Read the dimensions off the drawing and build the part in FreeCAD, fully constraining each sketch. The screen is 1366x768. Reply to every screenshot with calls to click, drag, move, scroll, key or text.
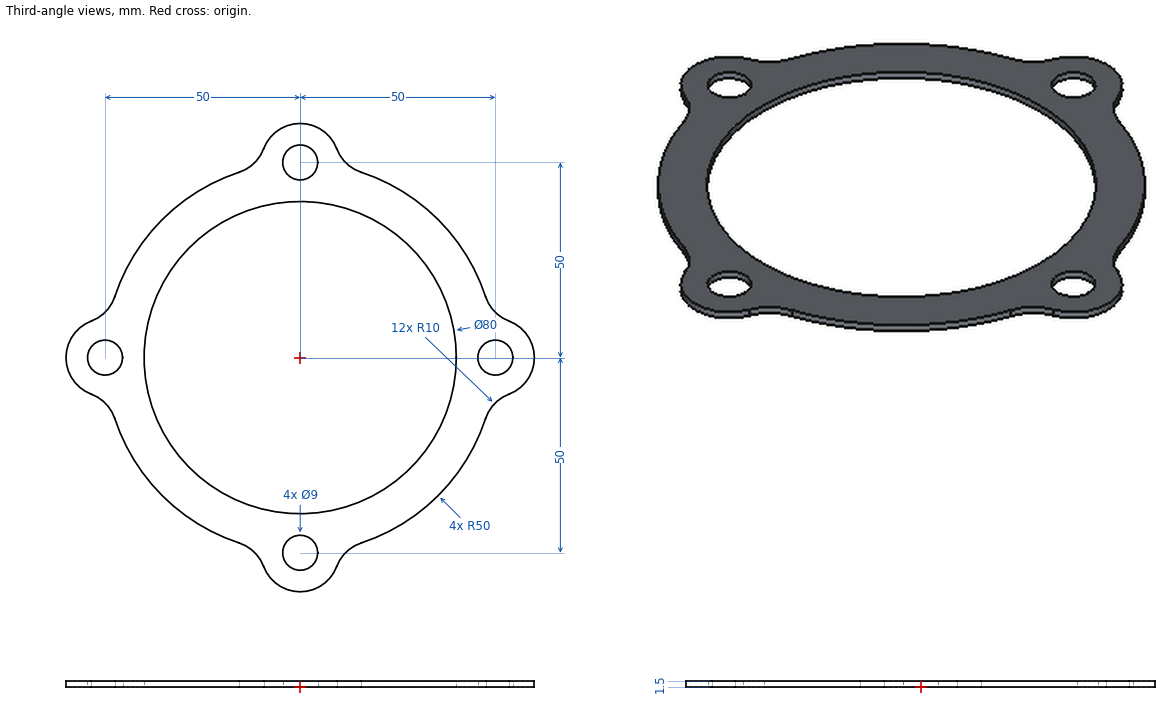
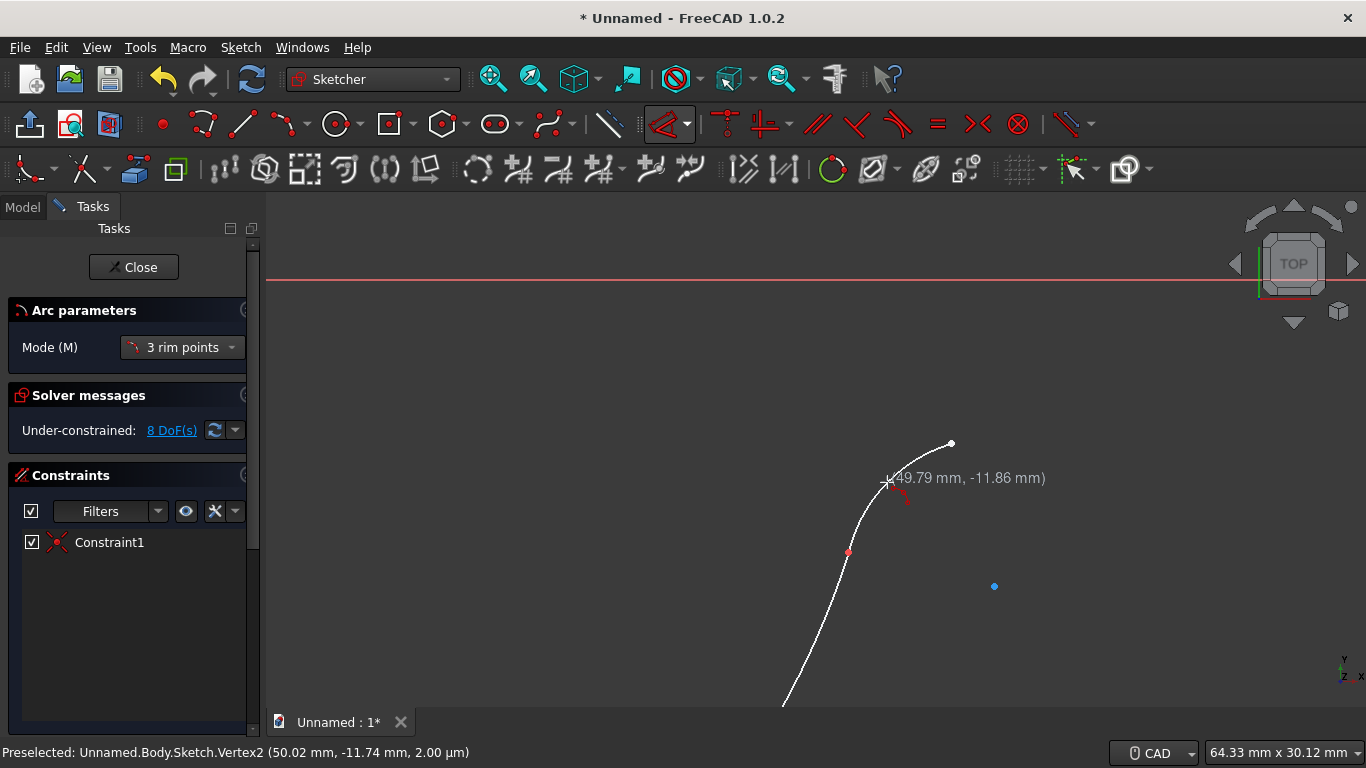
scroll(888, 483, down, 9)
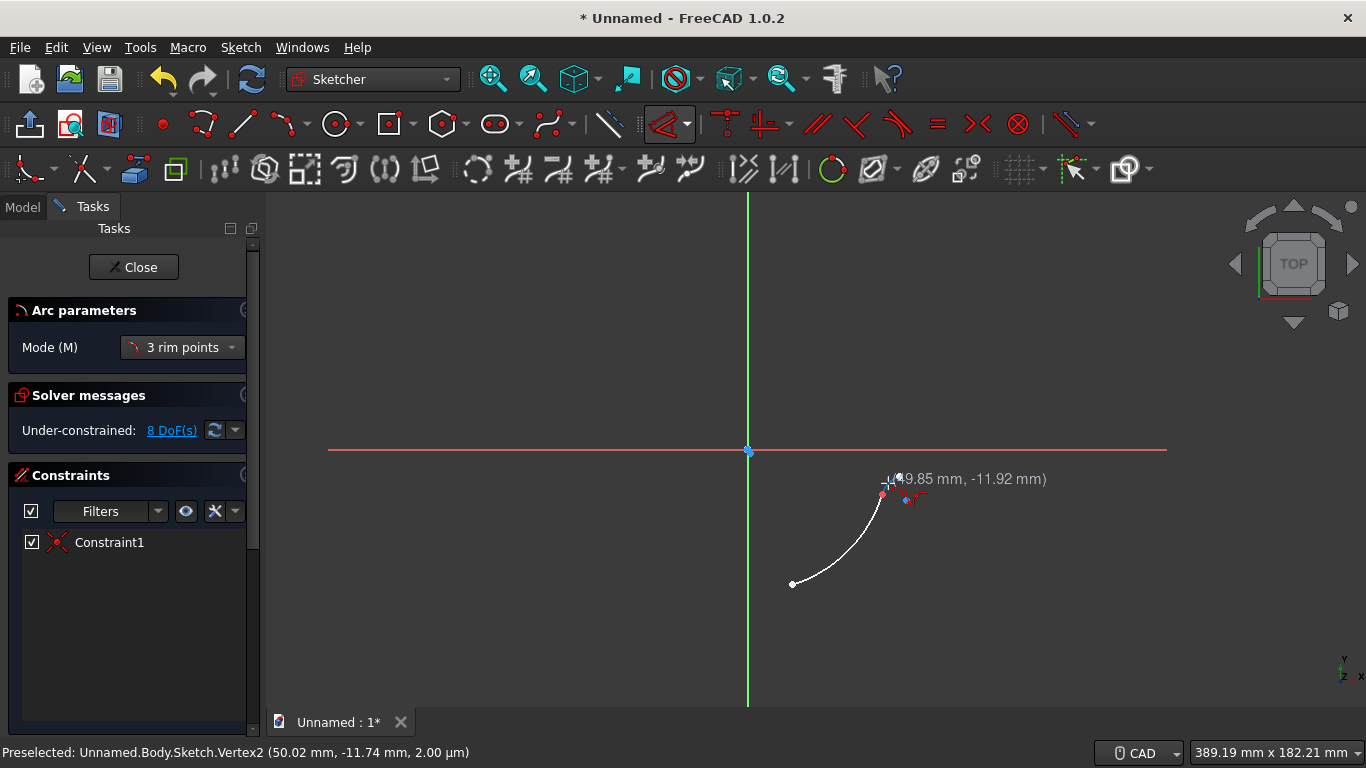
click(899, 477)
click(899, 423)
click(914, 463)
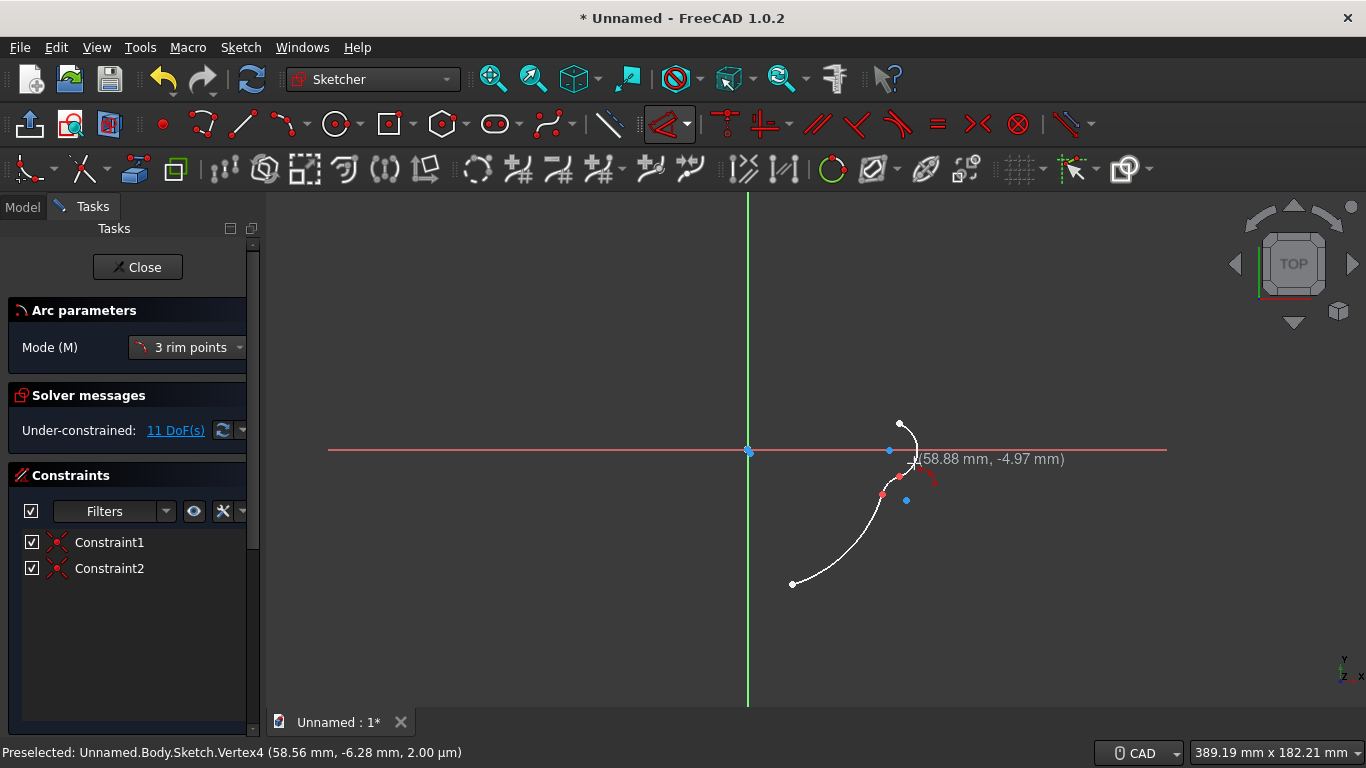
click(899, 424)
click(882, 406)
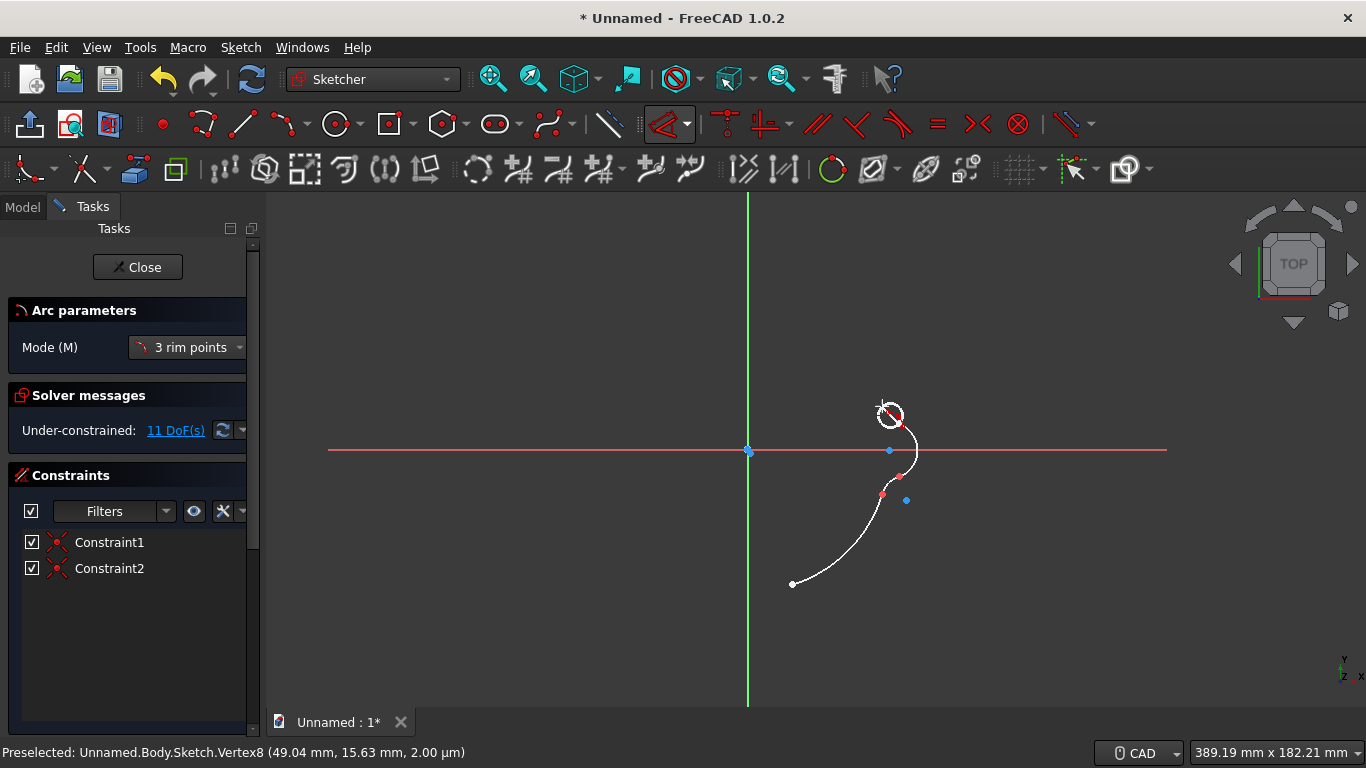
scroll(888, 417, up, 9)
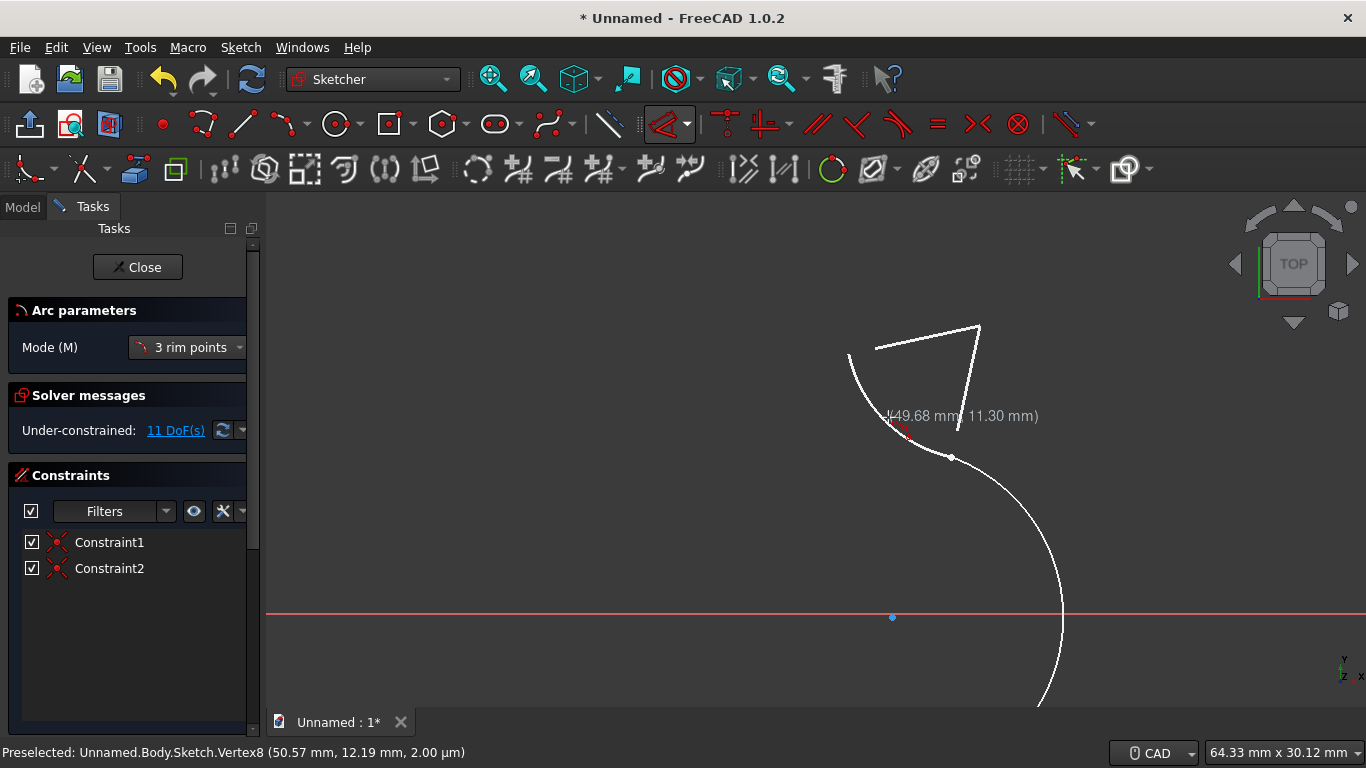
click(887, 412)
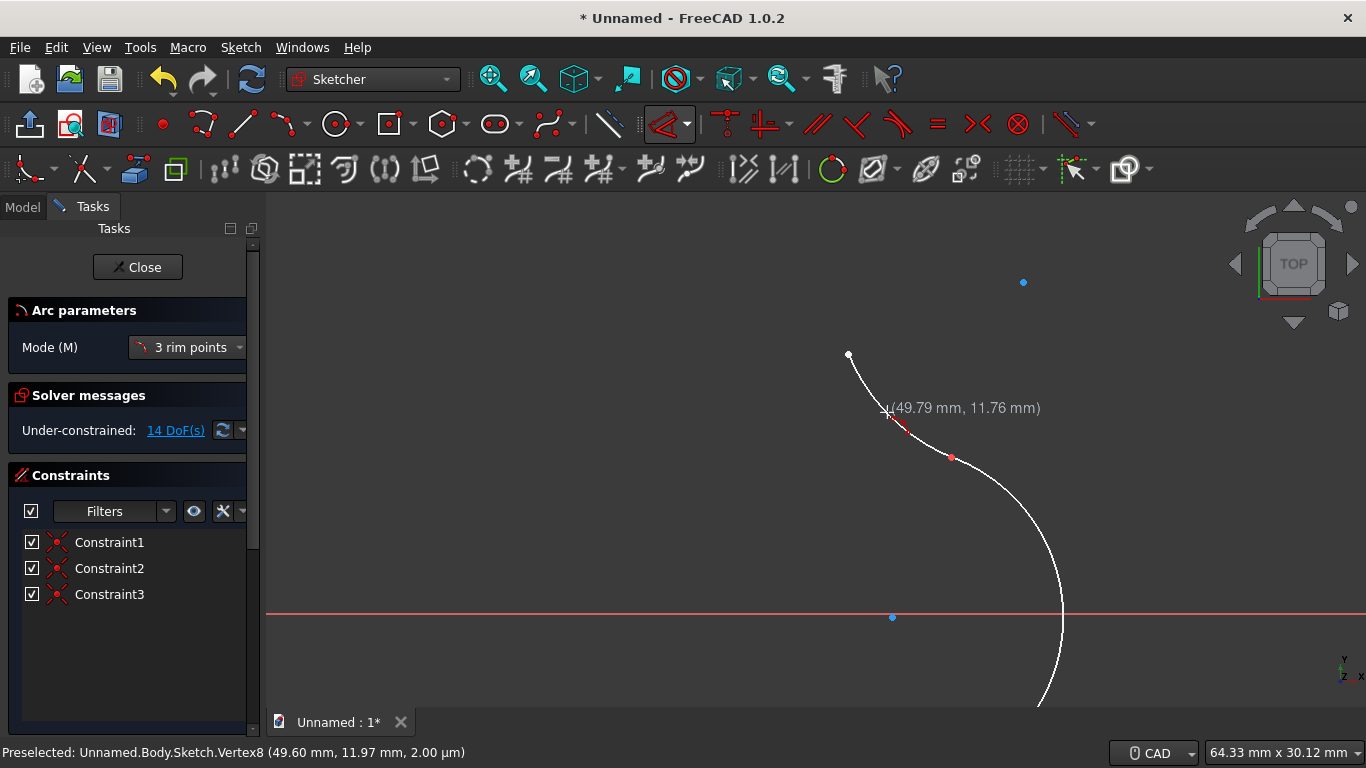
scroll(888, 417, down, 9)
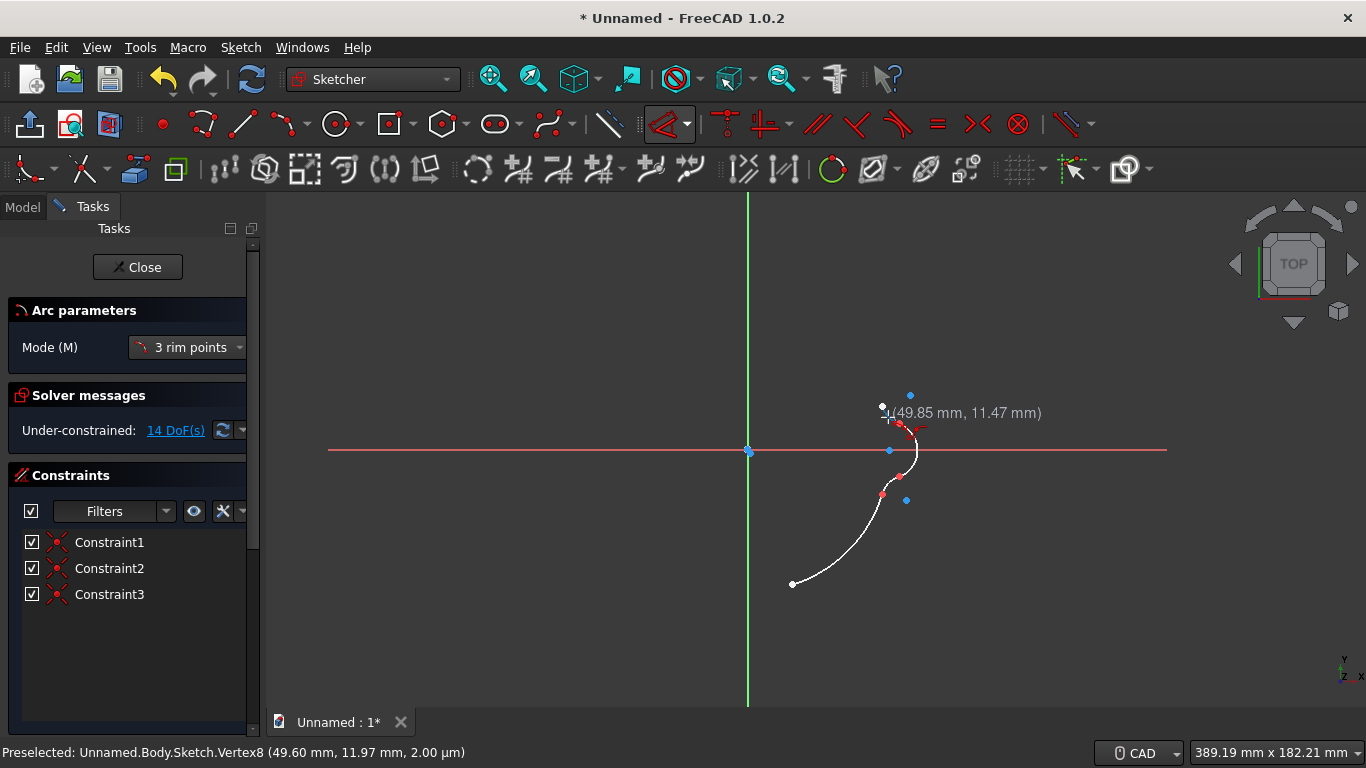
click(882, 407)
click(792, 316)
click(848, 350)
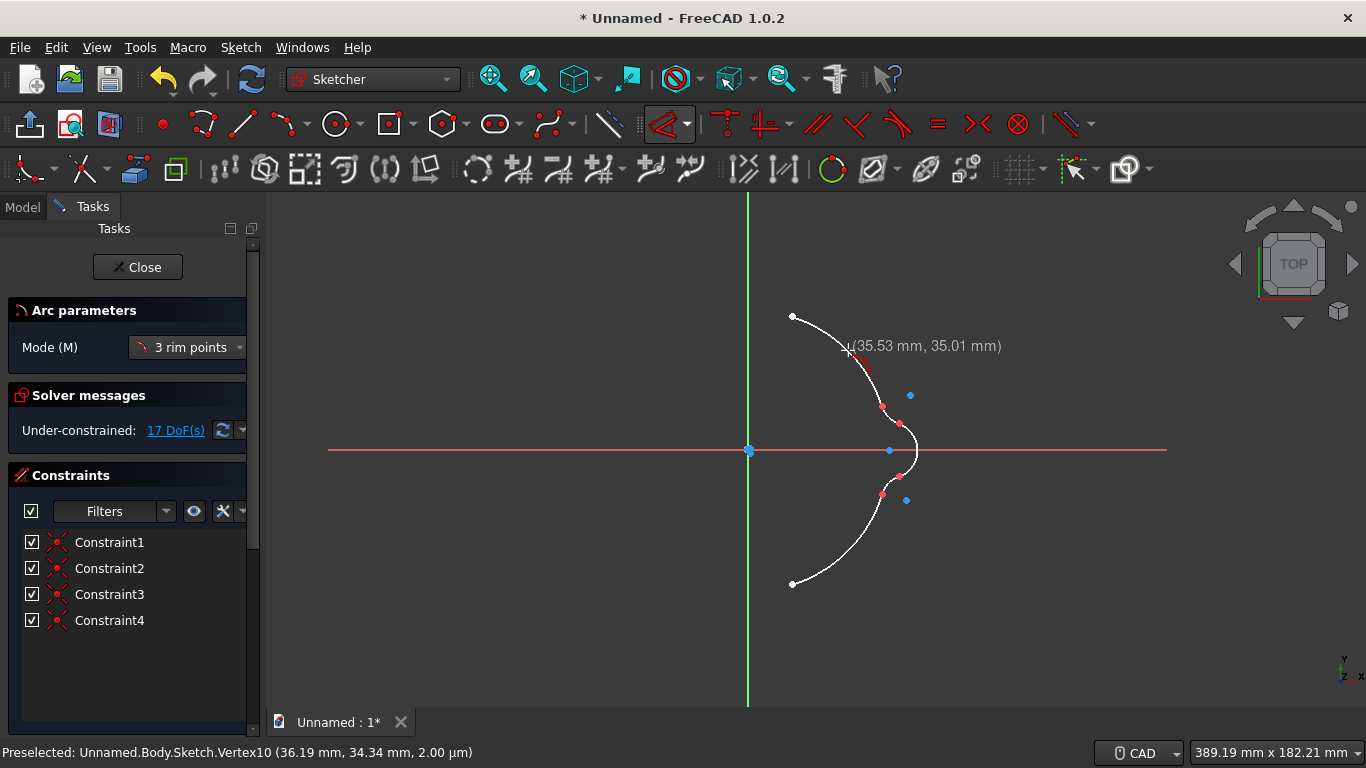
click(792, 317)
click(774, 299)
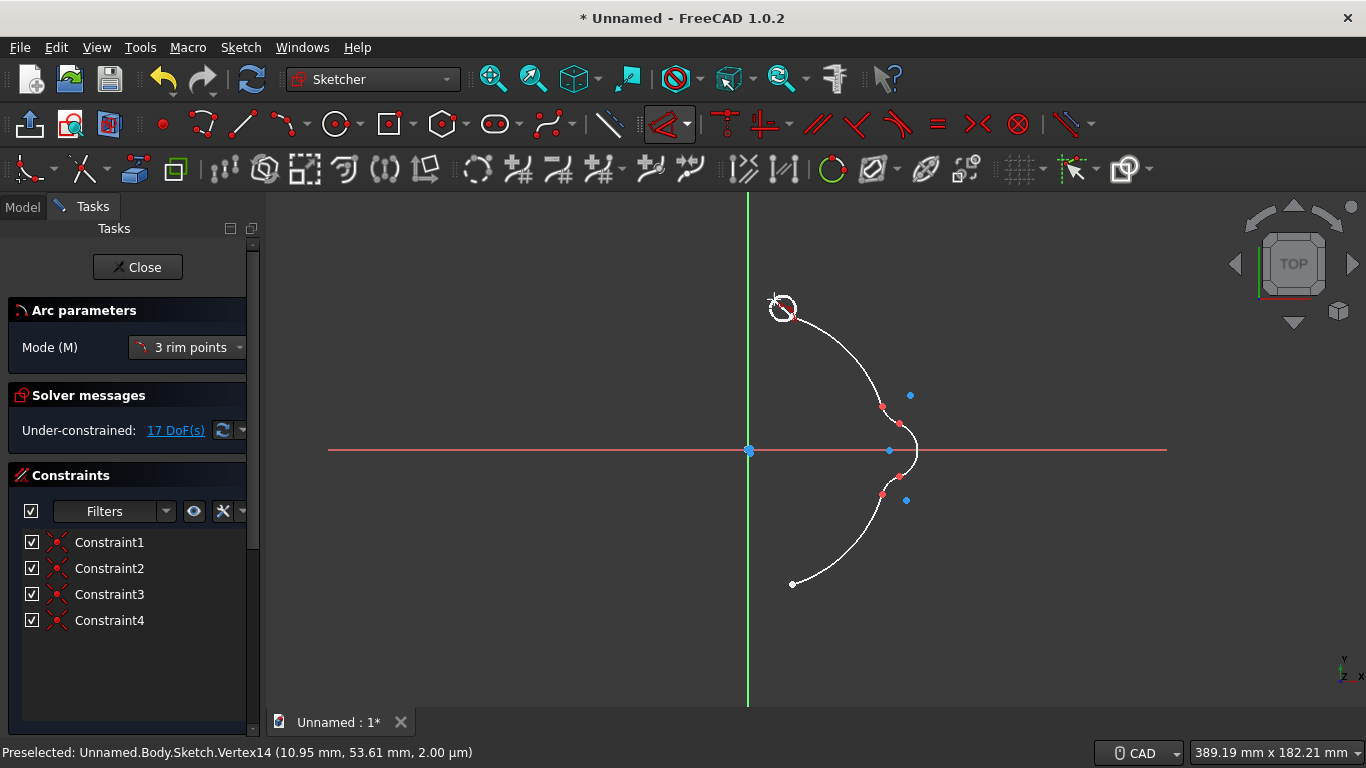
scroll(781, 309, up, 9)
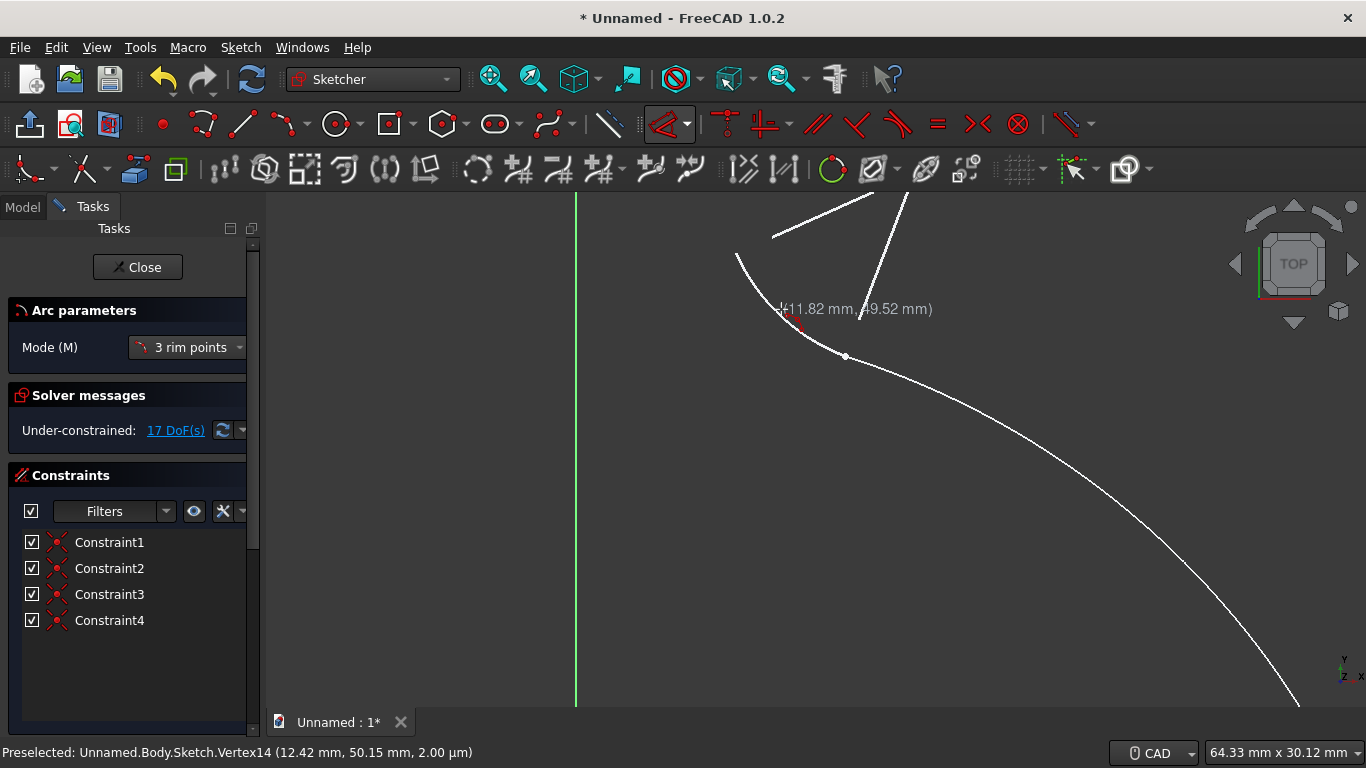
click(778, 309)